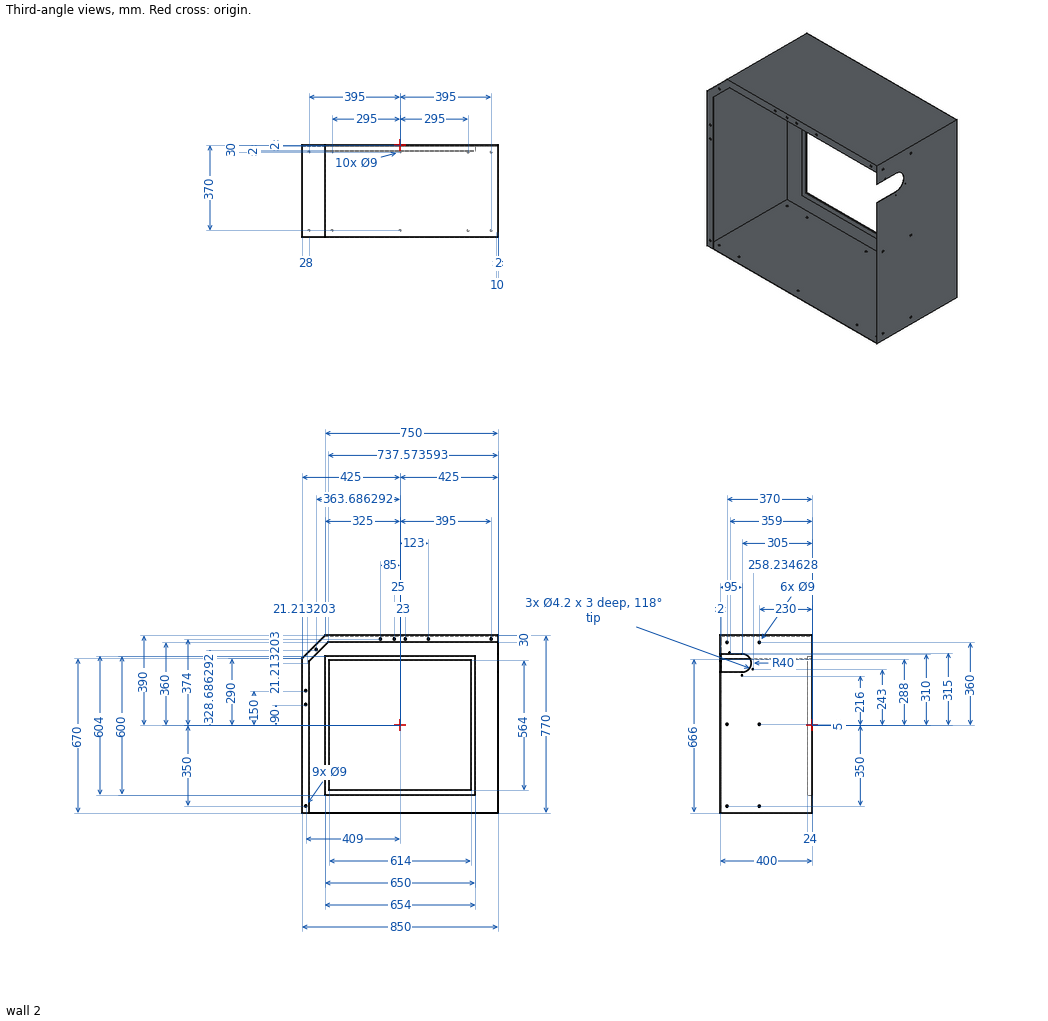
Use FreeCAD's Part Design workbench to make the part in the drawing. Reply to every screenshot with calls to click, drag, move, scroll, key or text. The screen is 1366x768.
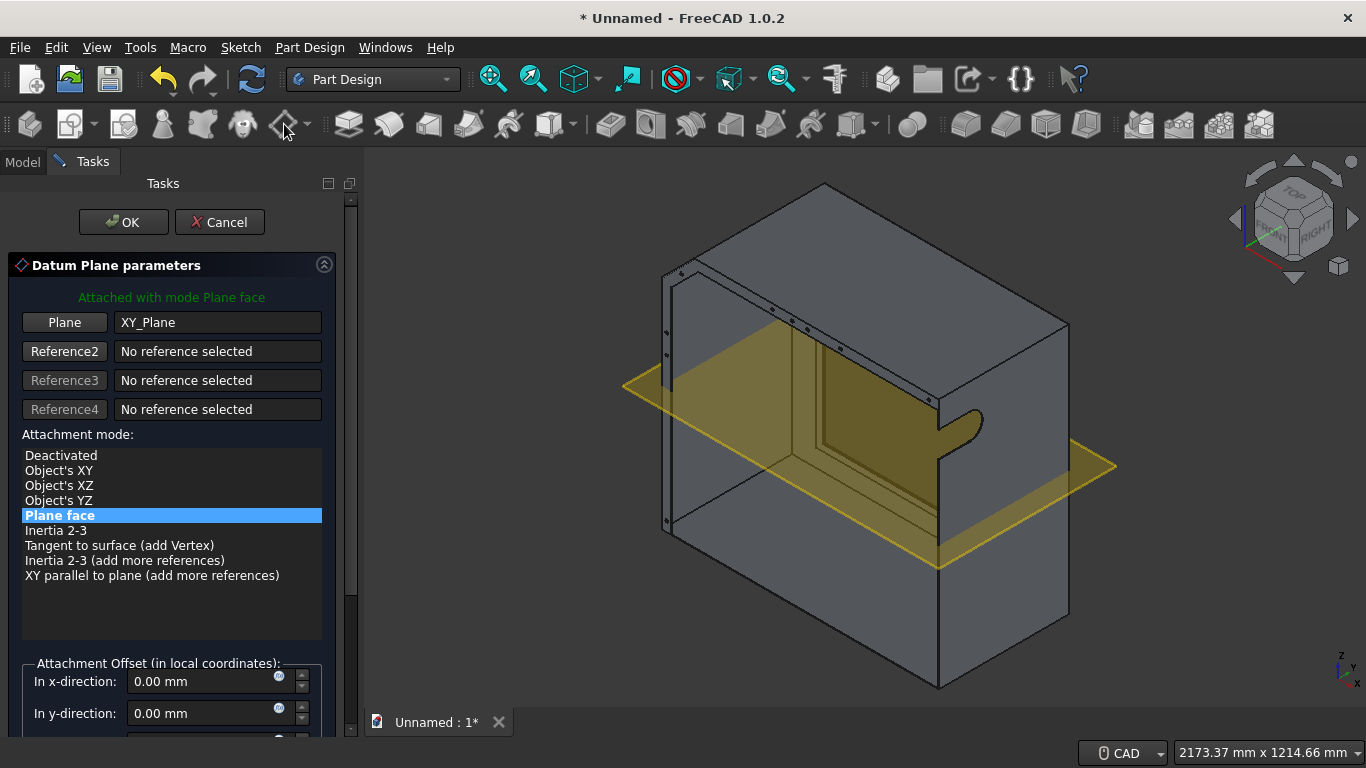
scroll(351, 464, down, 2)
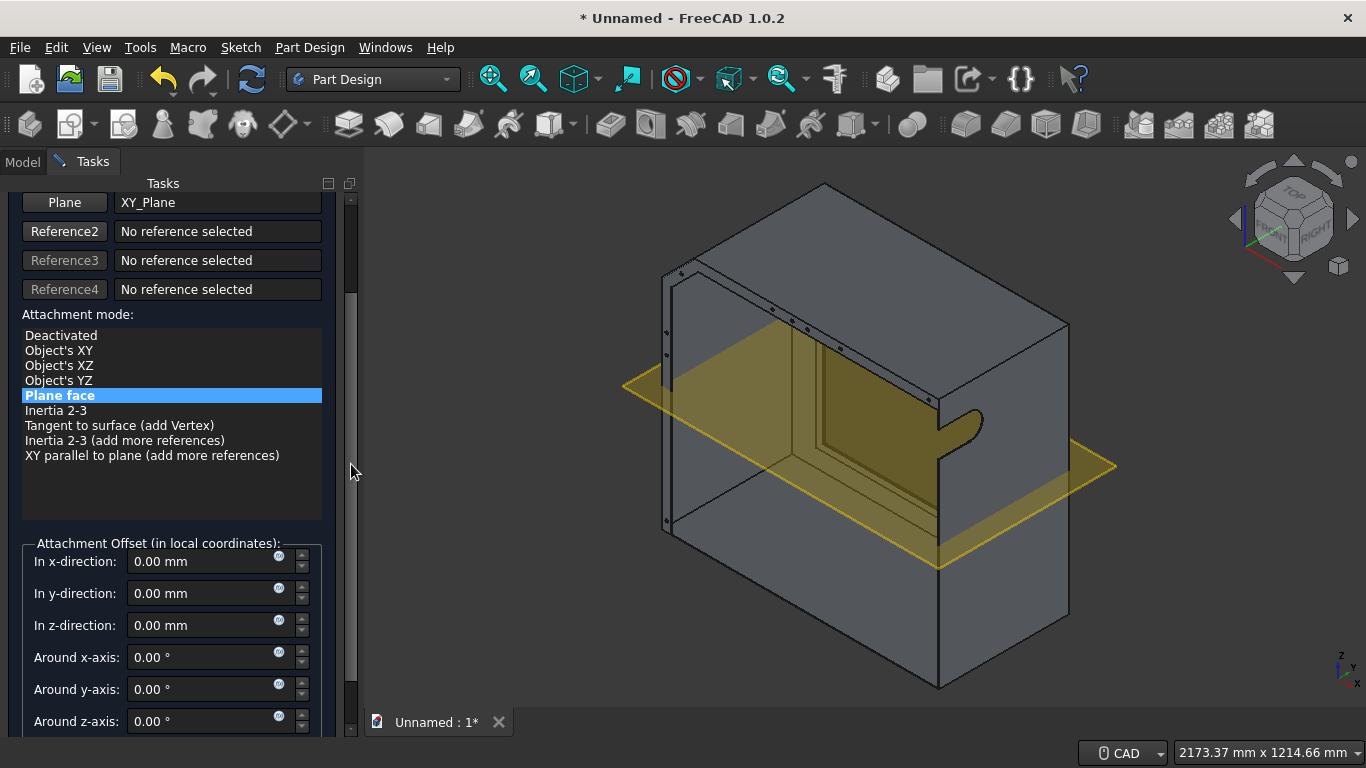
triple_click(210, 625)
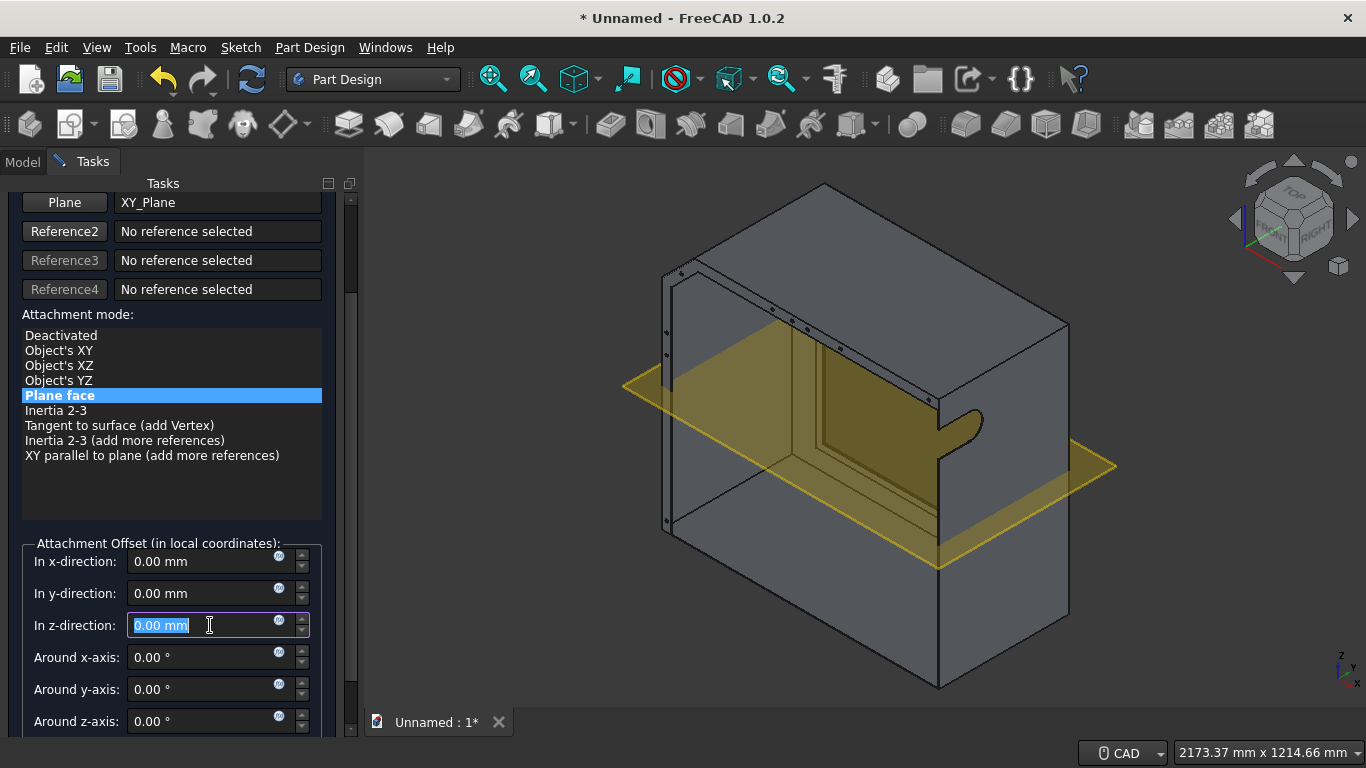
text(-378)
key(Tab)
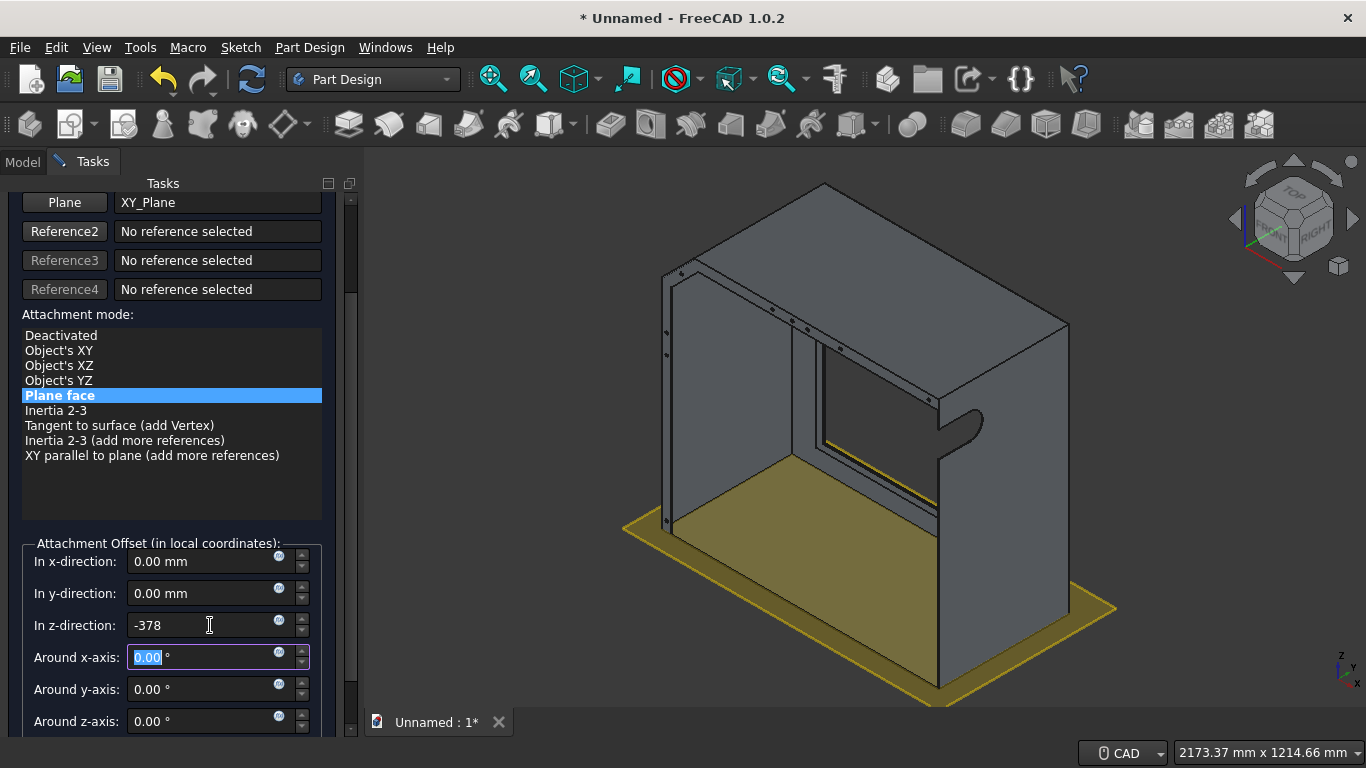
scroll(351, 464, up, 3)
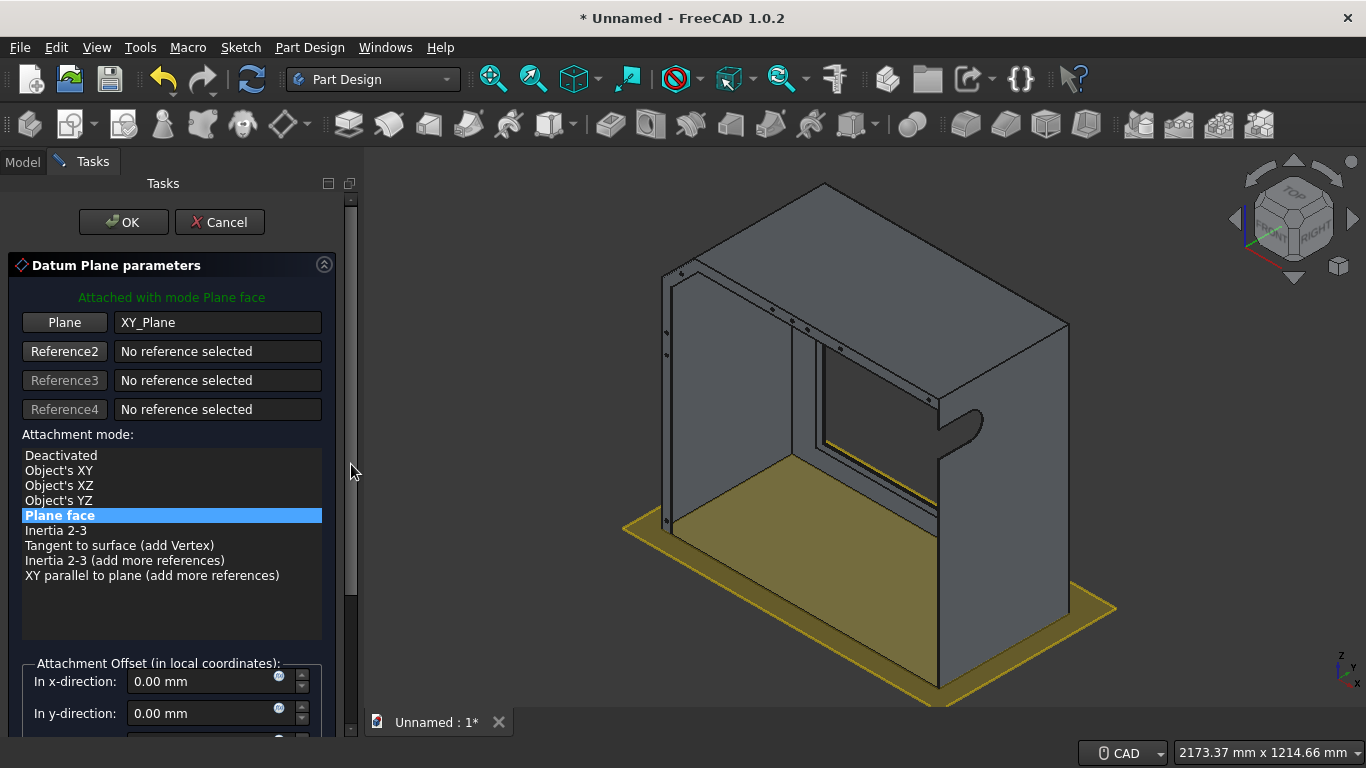
click(124, 222)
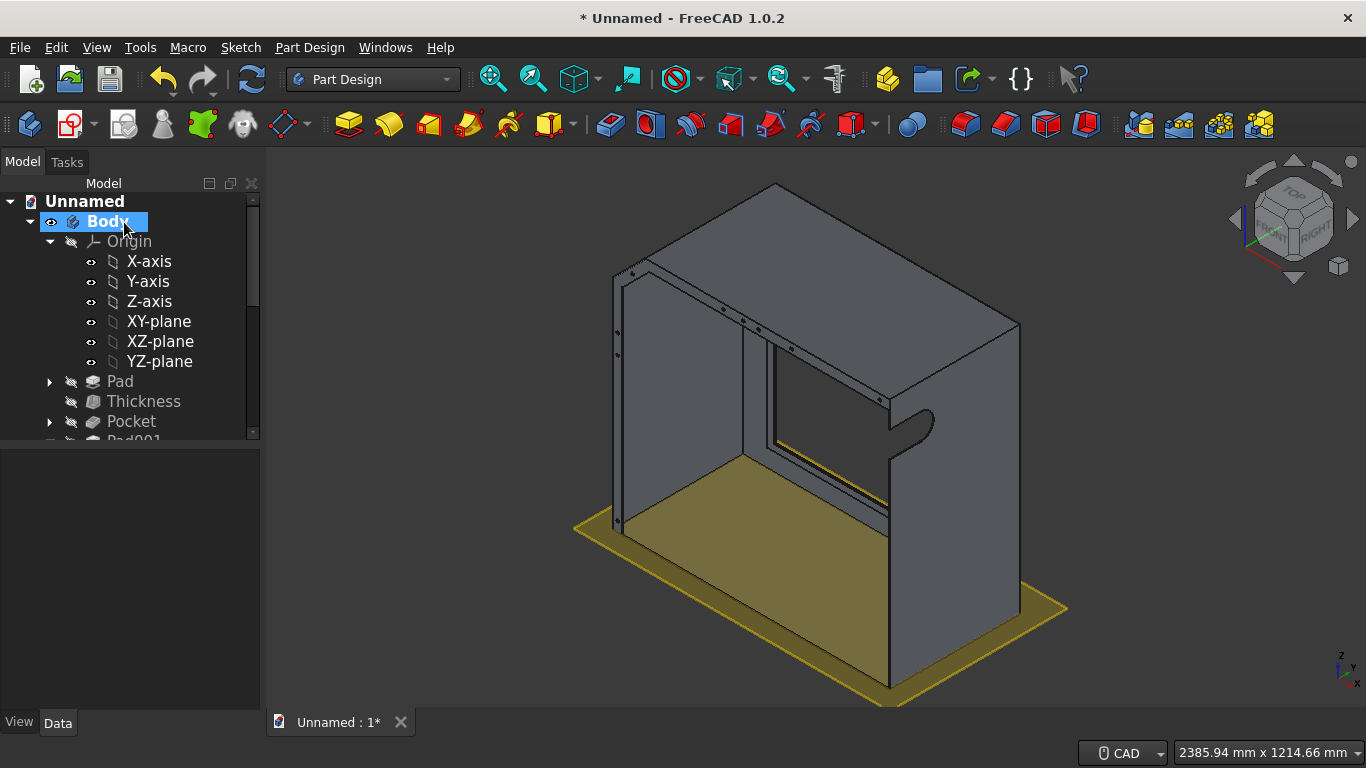
scroll(100, 317, down, 3)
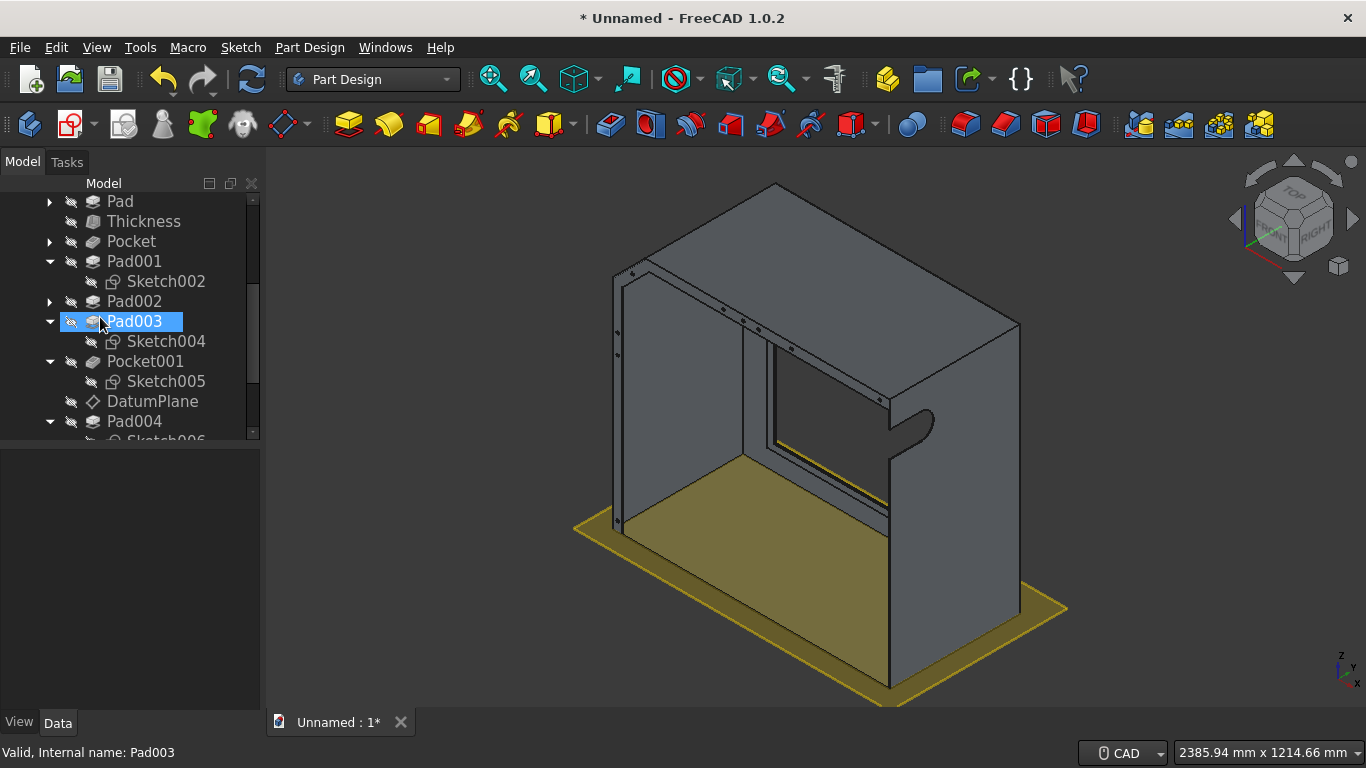
scroll(140, 317, up, 15)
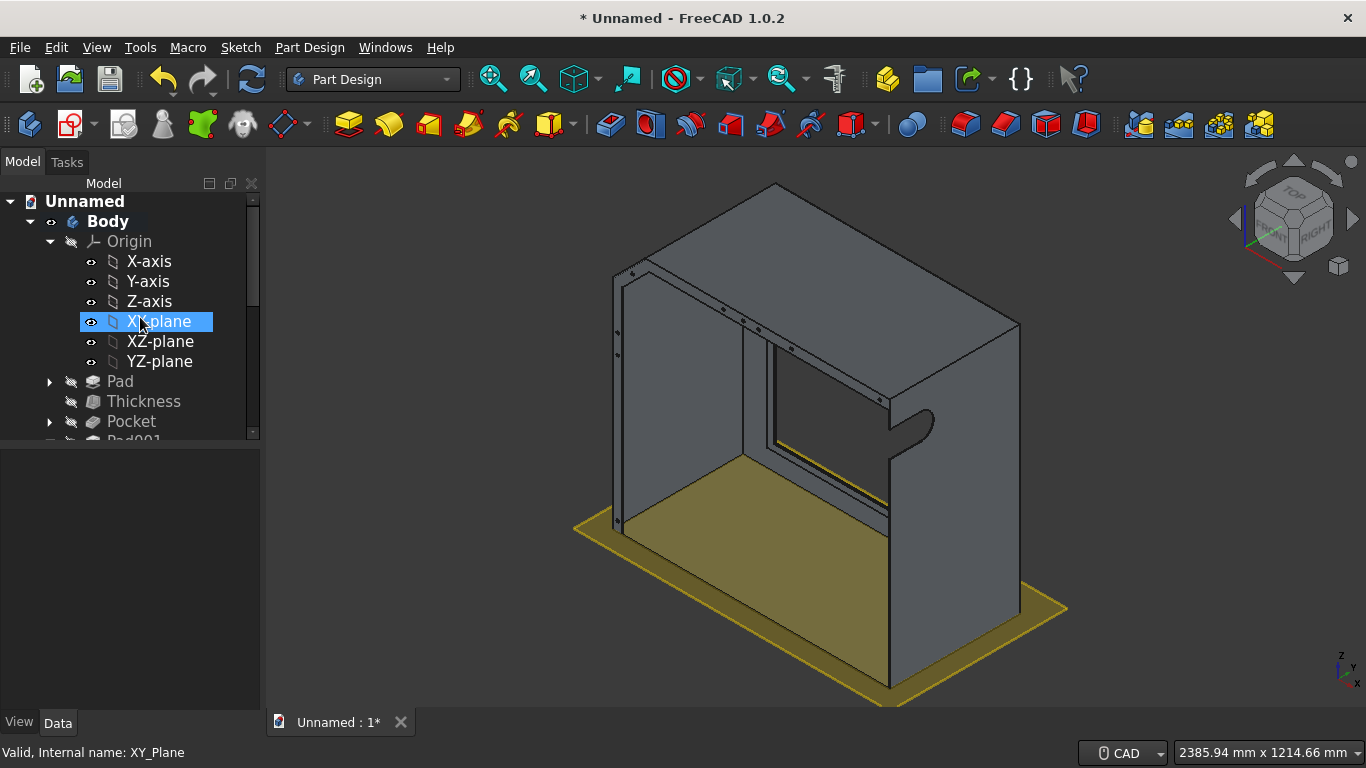
scroll(100, 317, down, 6)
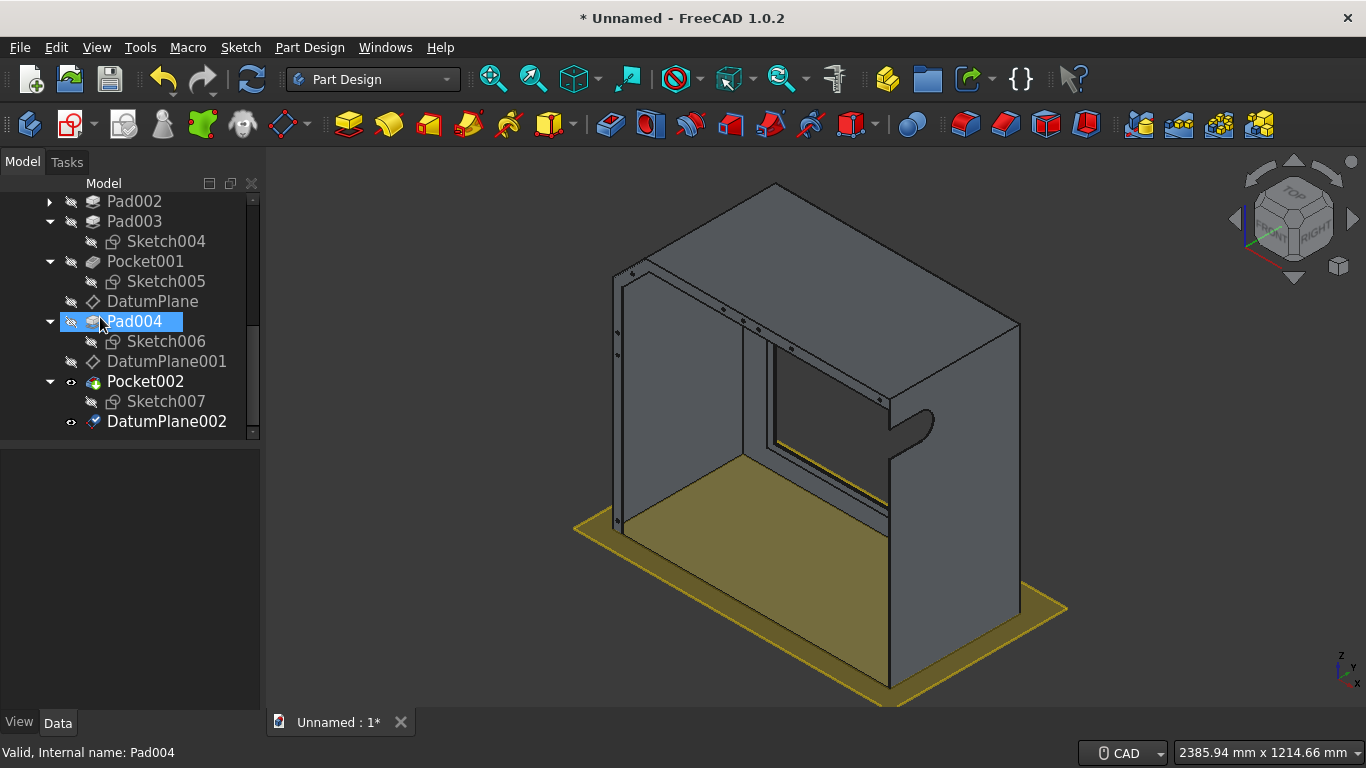
click(116, 422)